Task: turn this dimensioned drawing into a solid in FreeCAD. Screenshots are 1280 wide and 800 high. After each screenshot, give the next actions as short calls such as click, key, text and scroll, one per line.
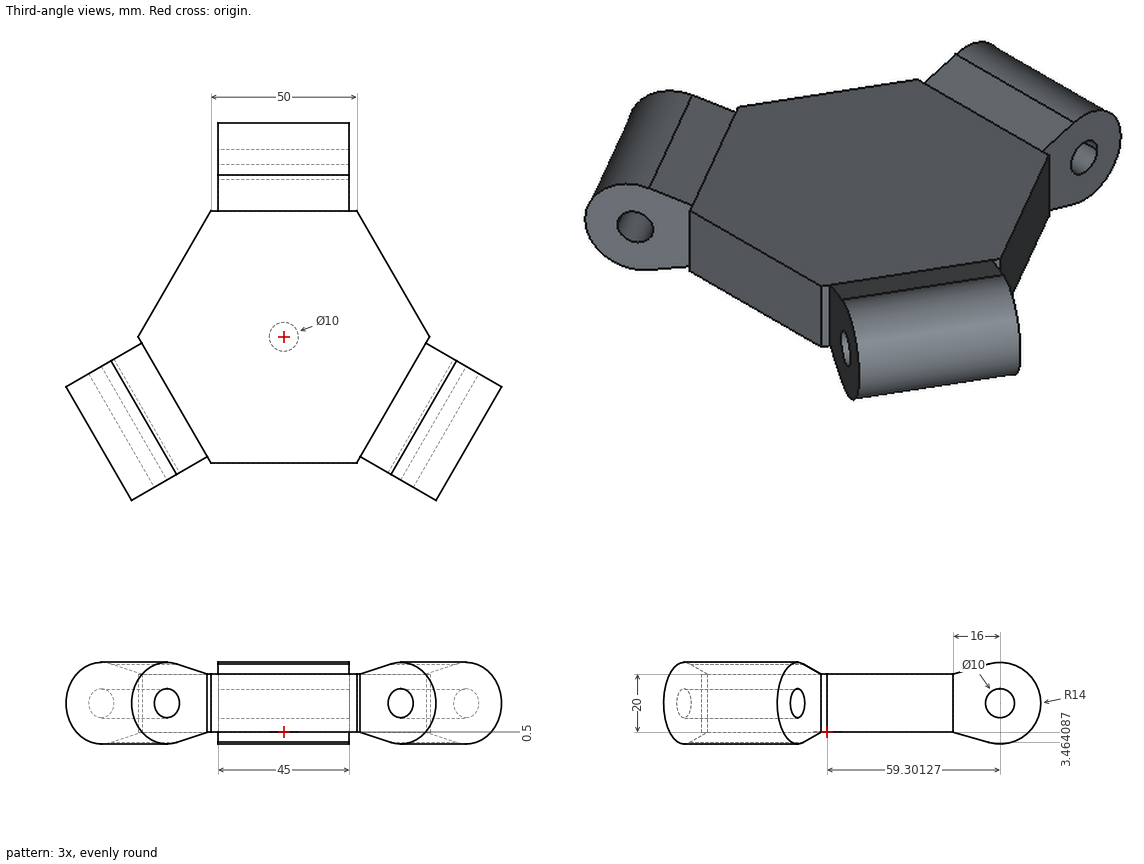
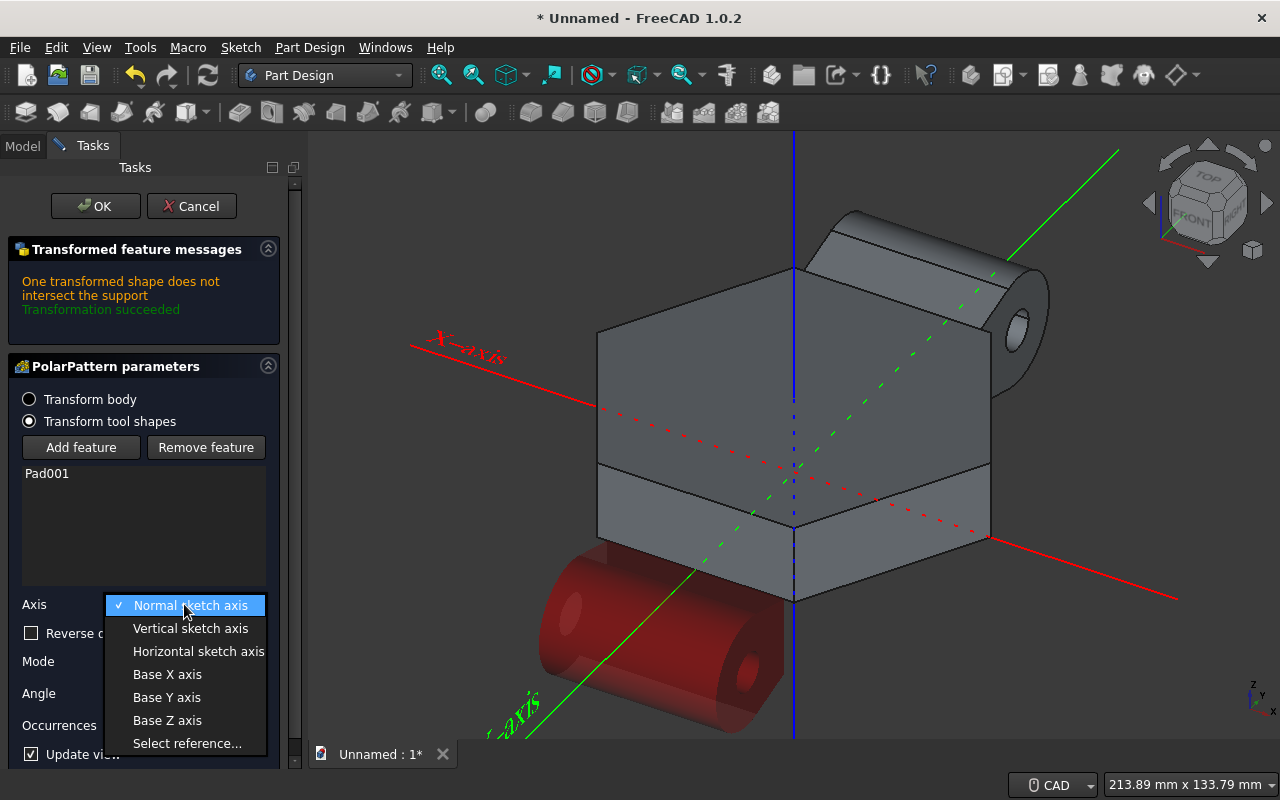
click(184, 720)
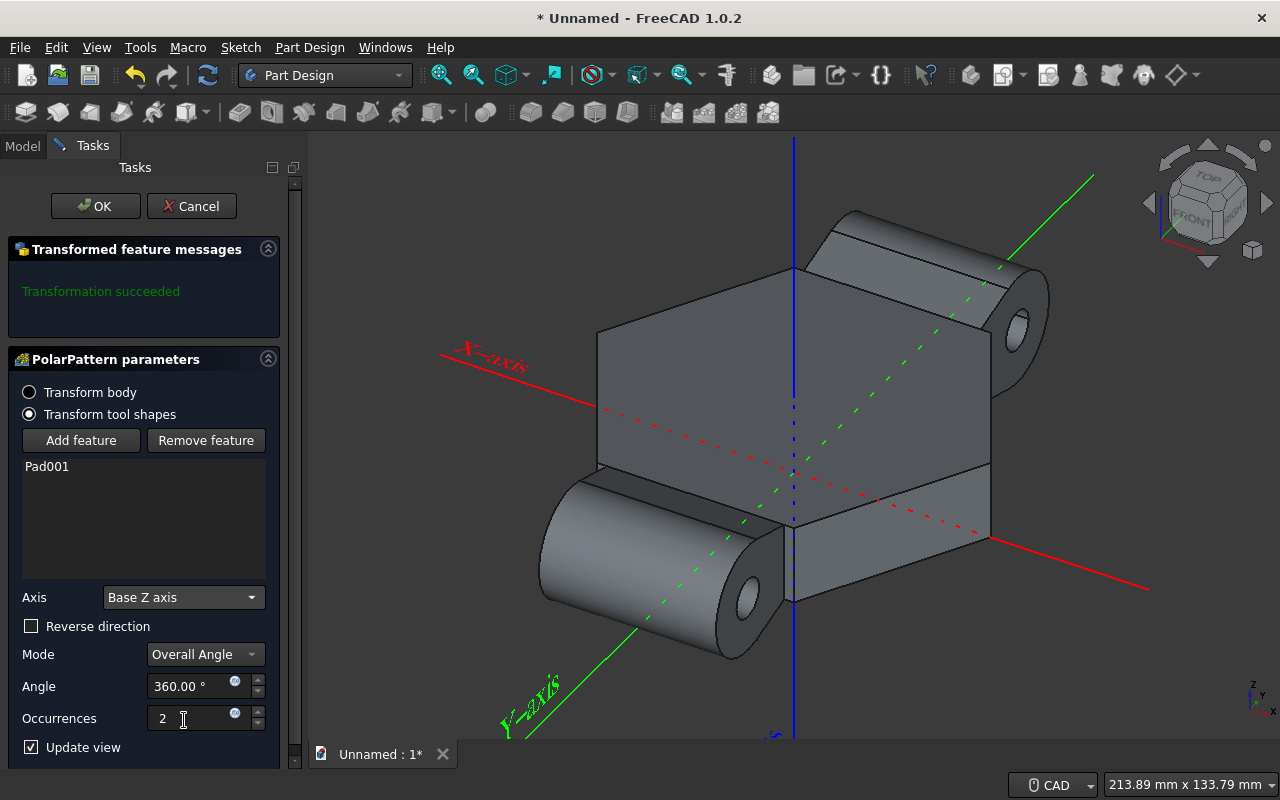
triple_click(198, 718)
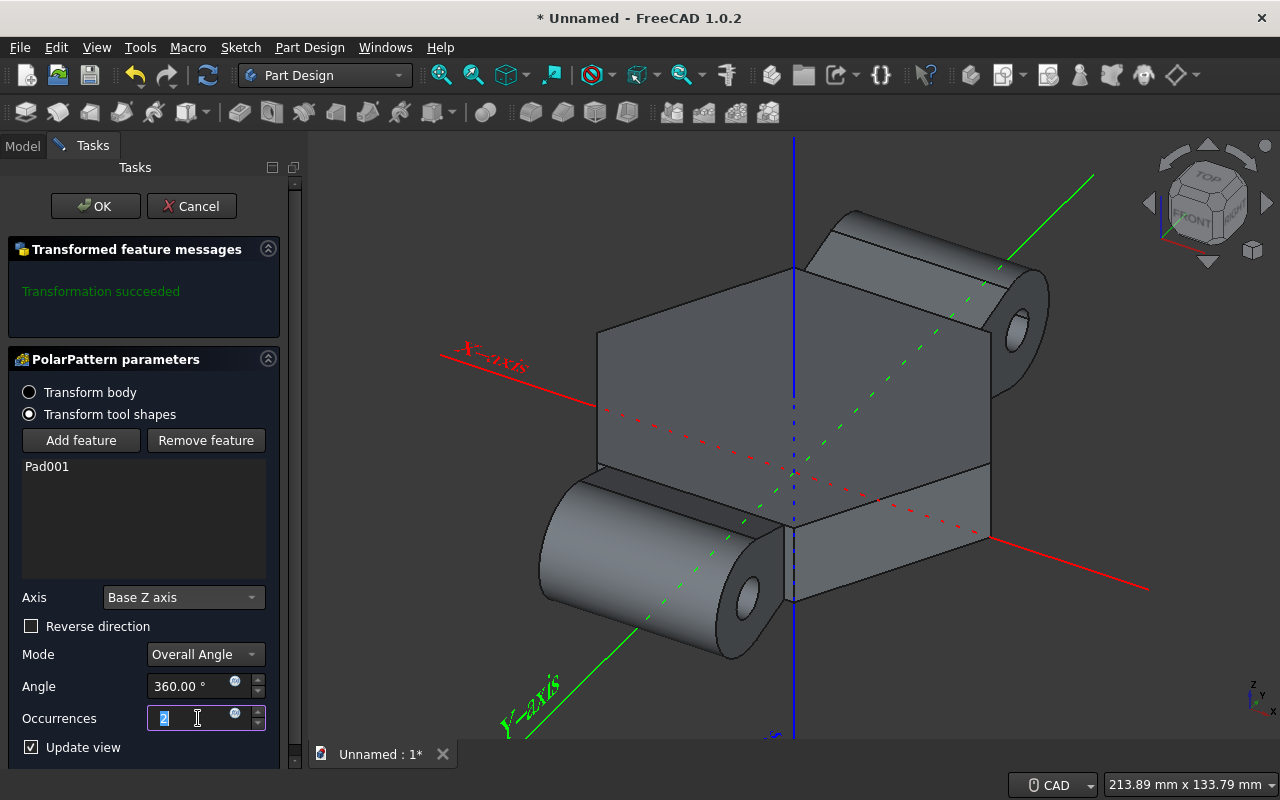
text(3)
key(Tab)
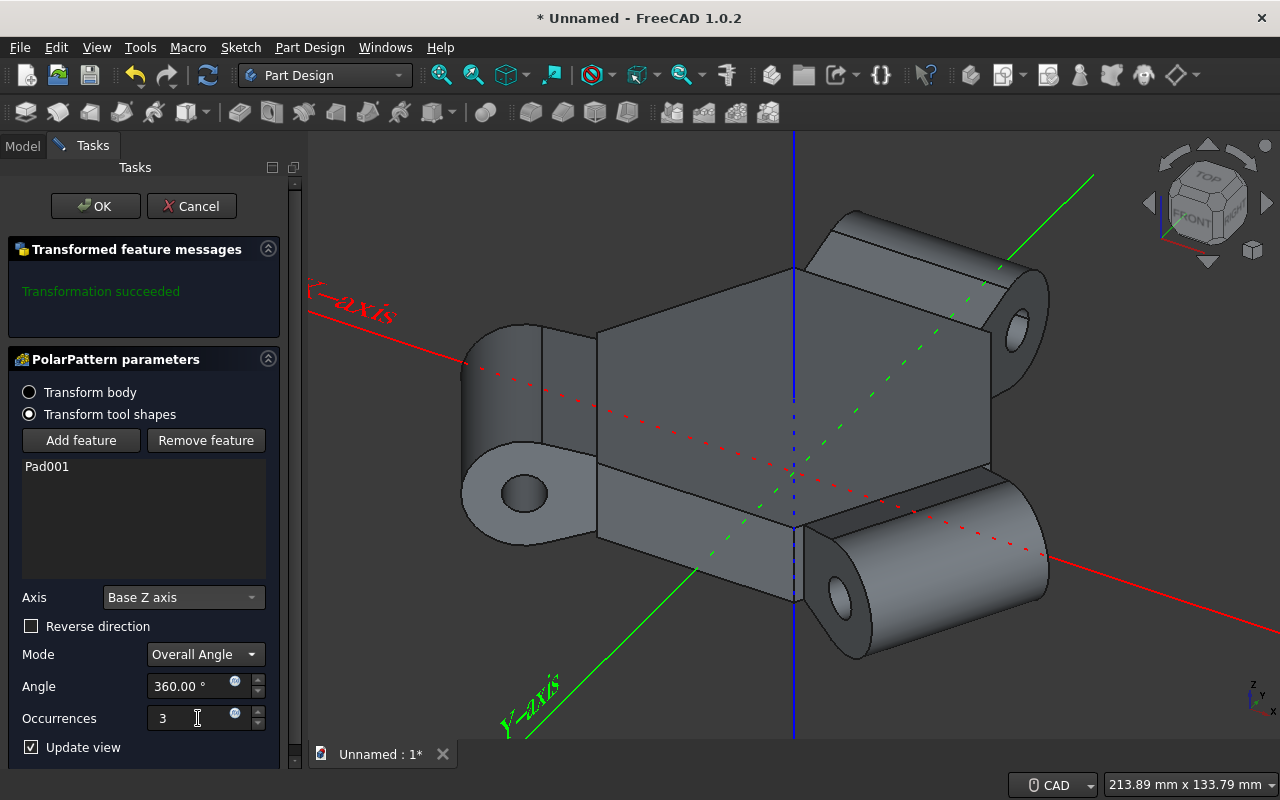
click(96, 206)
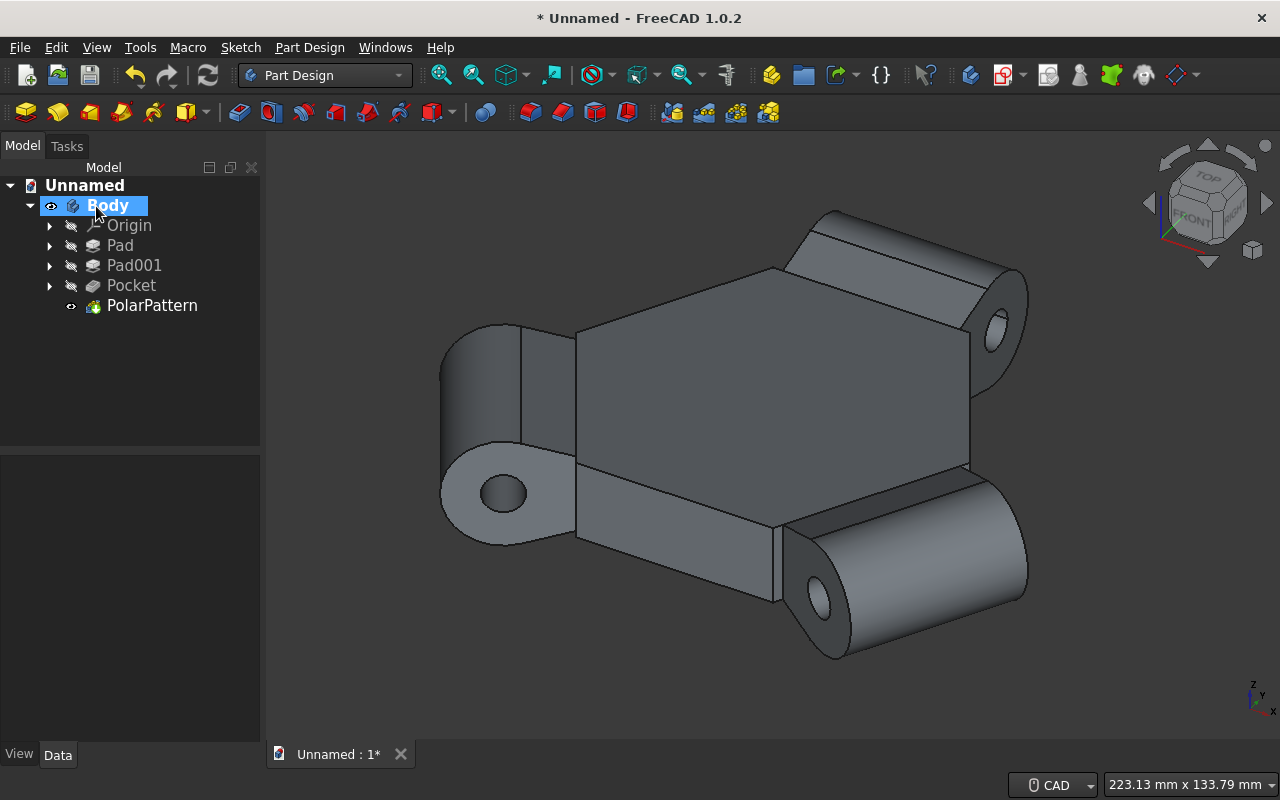
key(0)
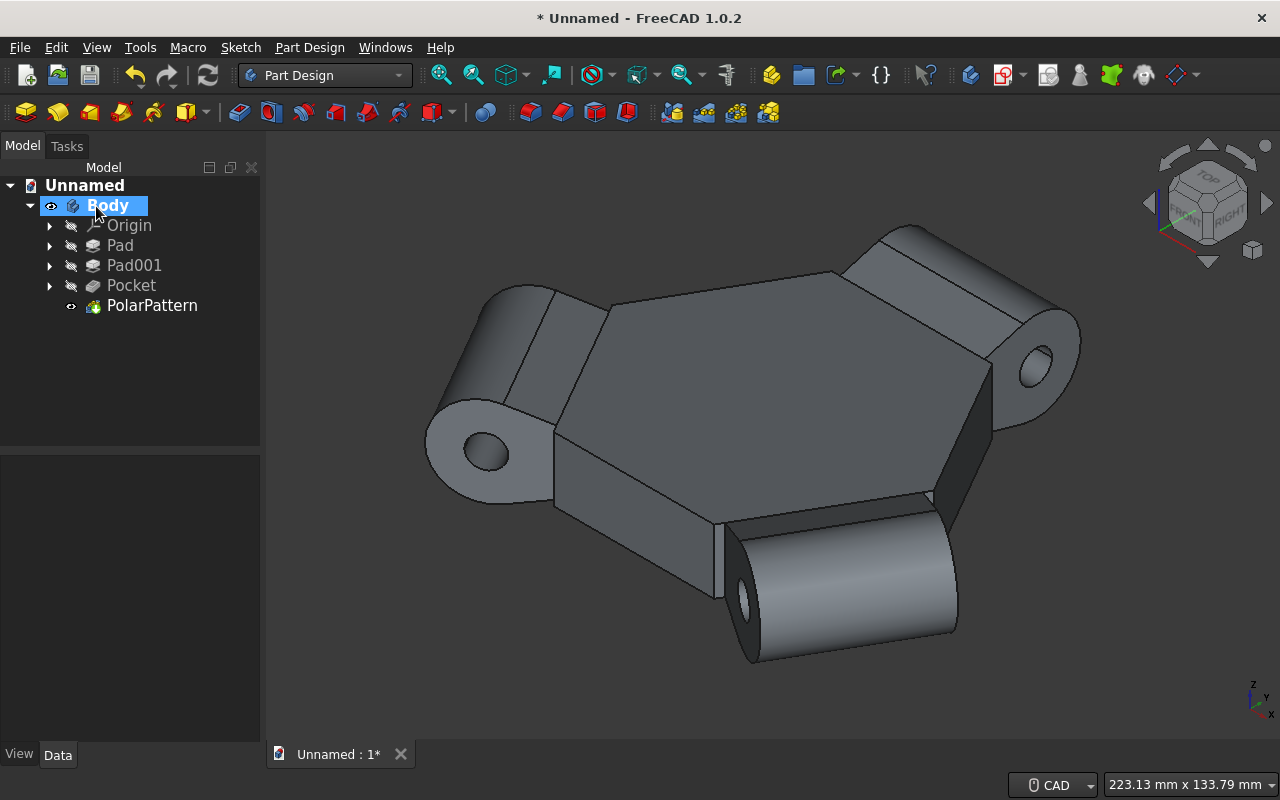
click(442, 76)